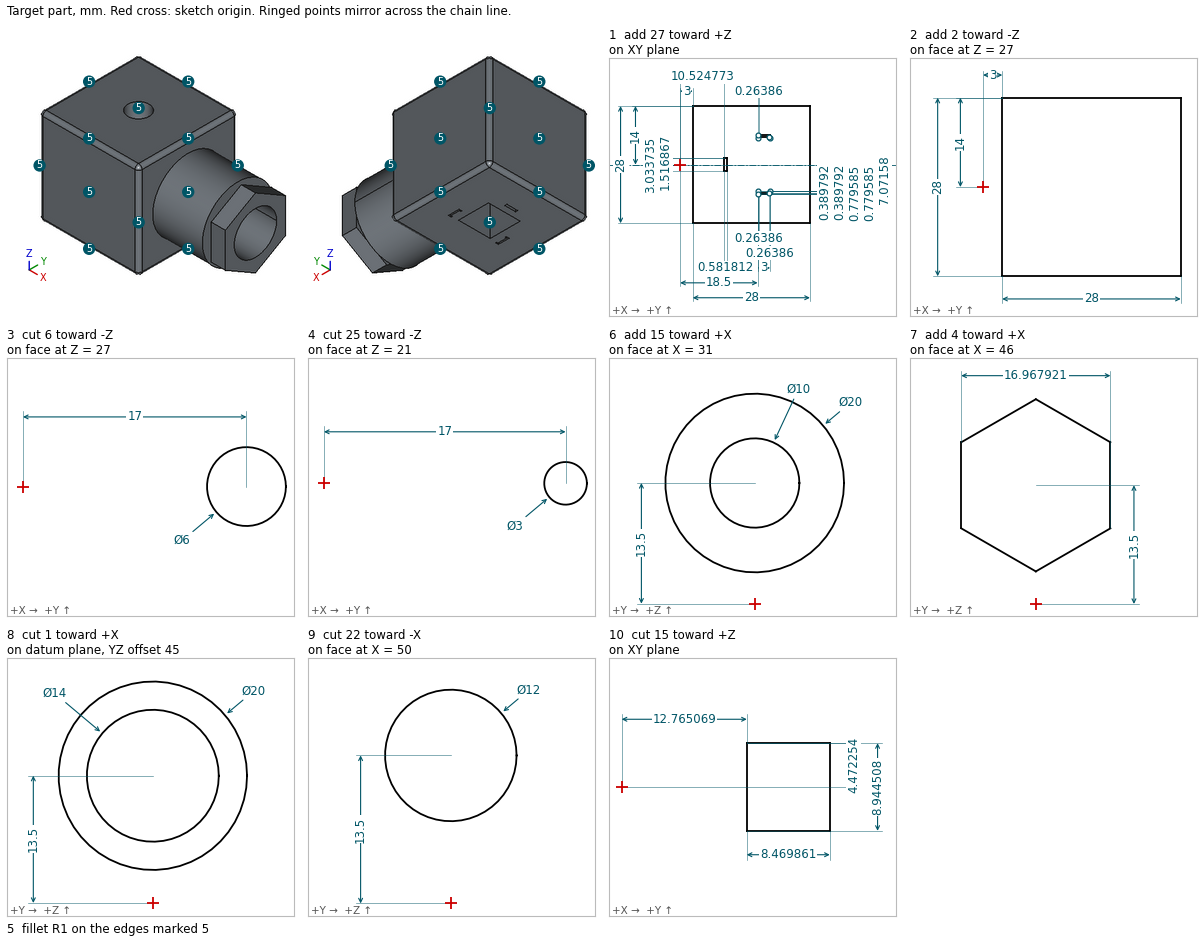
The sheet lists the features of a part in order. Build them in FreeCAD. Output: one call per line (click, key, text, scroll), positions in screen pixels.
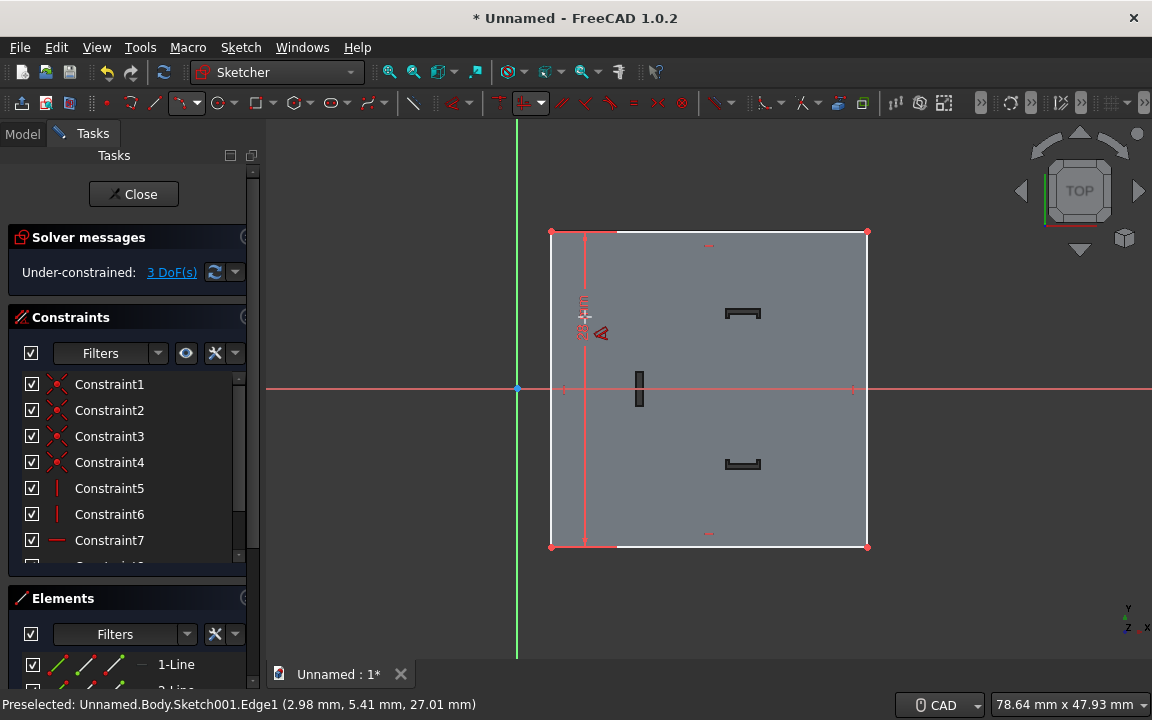
click(646, 547)
click(709, 581)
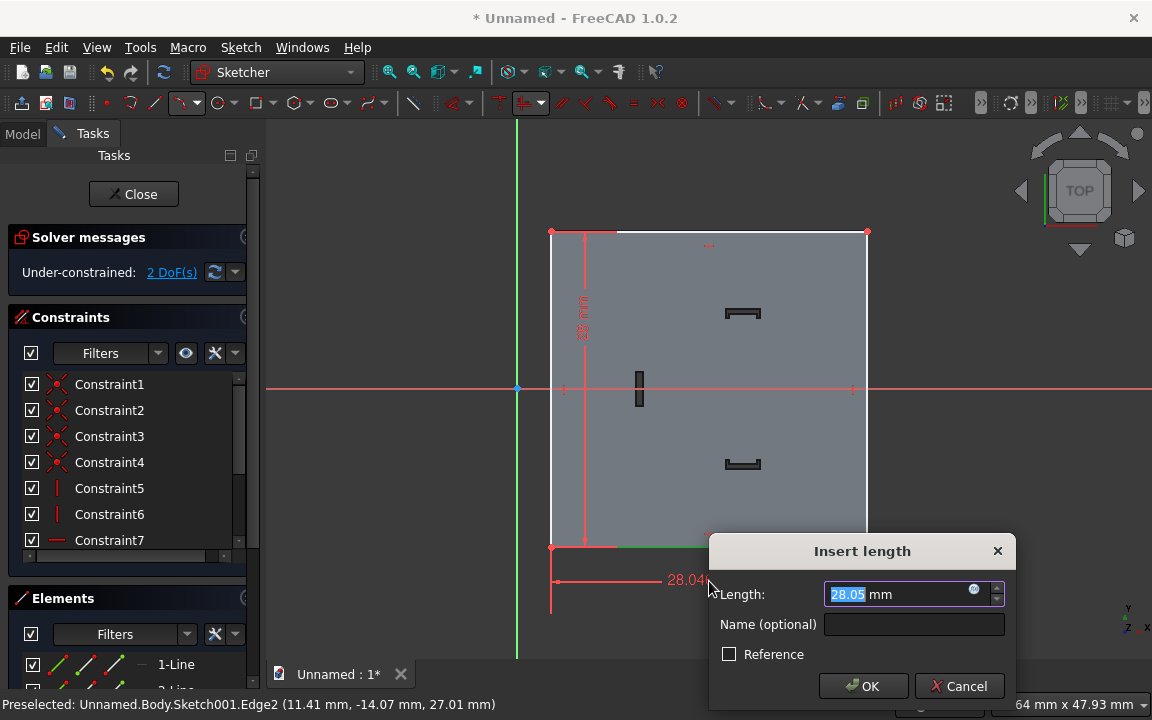
text(28)
key(Return)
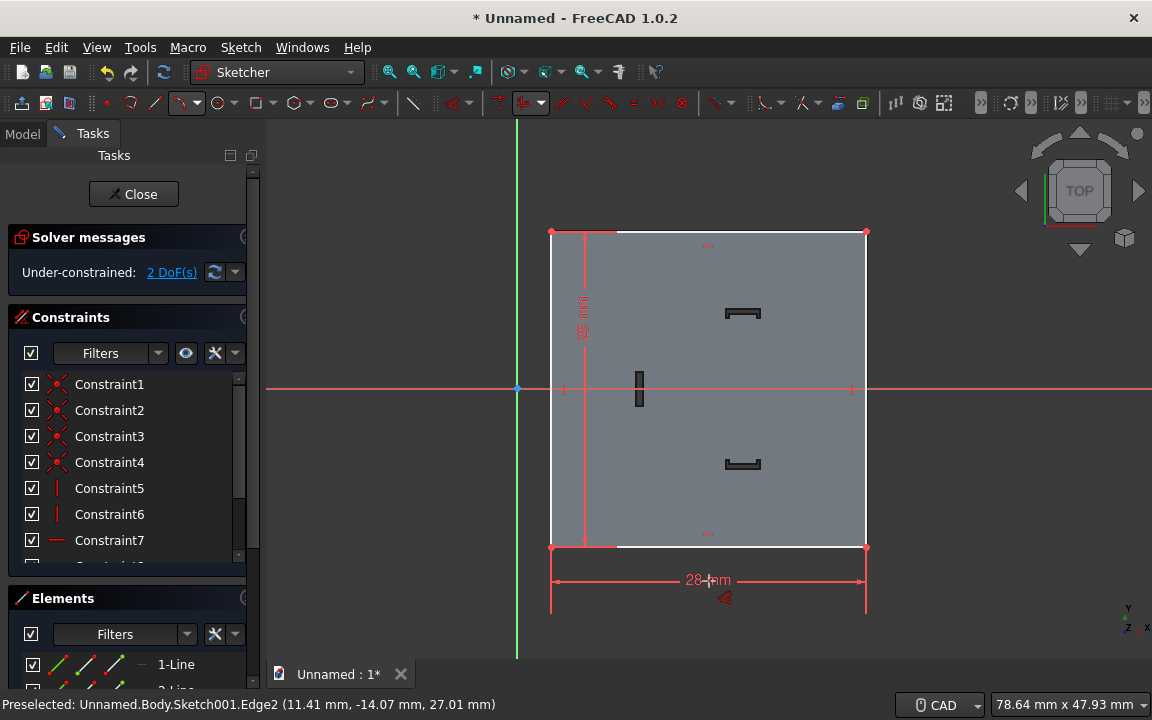
click(551, 232)
click(534, 198)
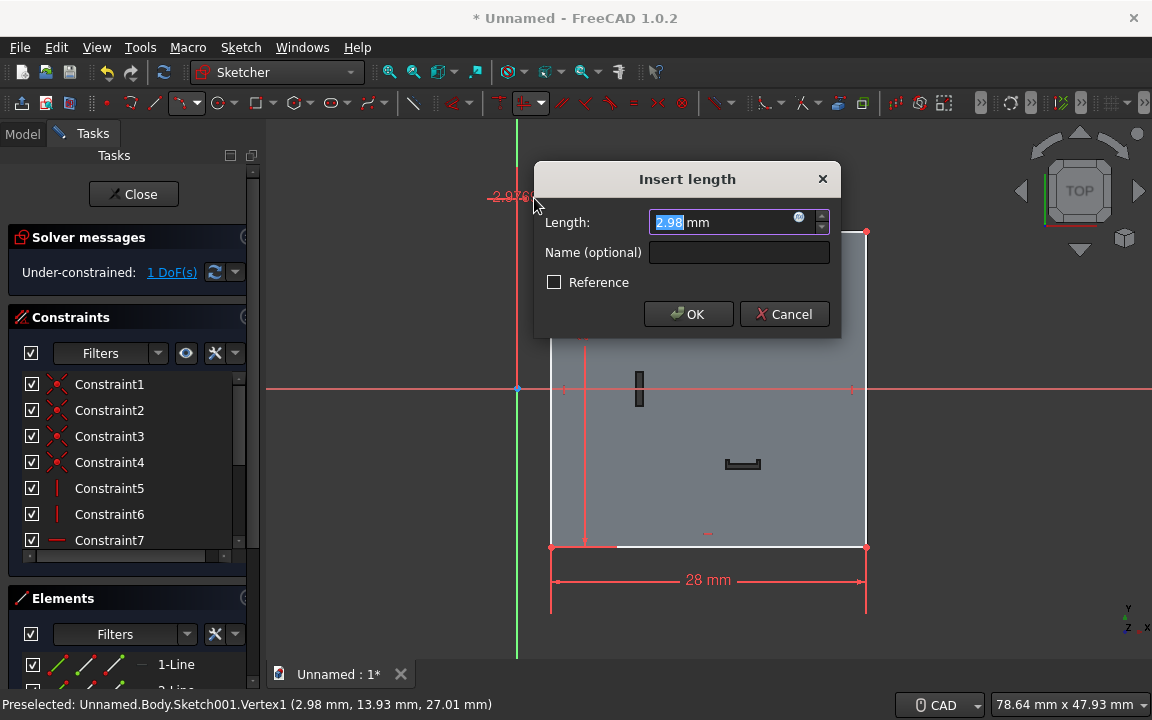
text(3)
key(Return)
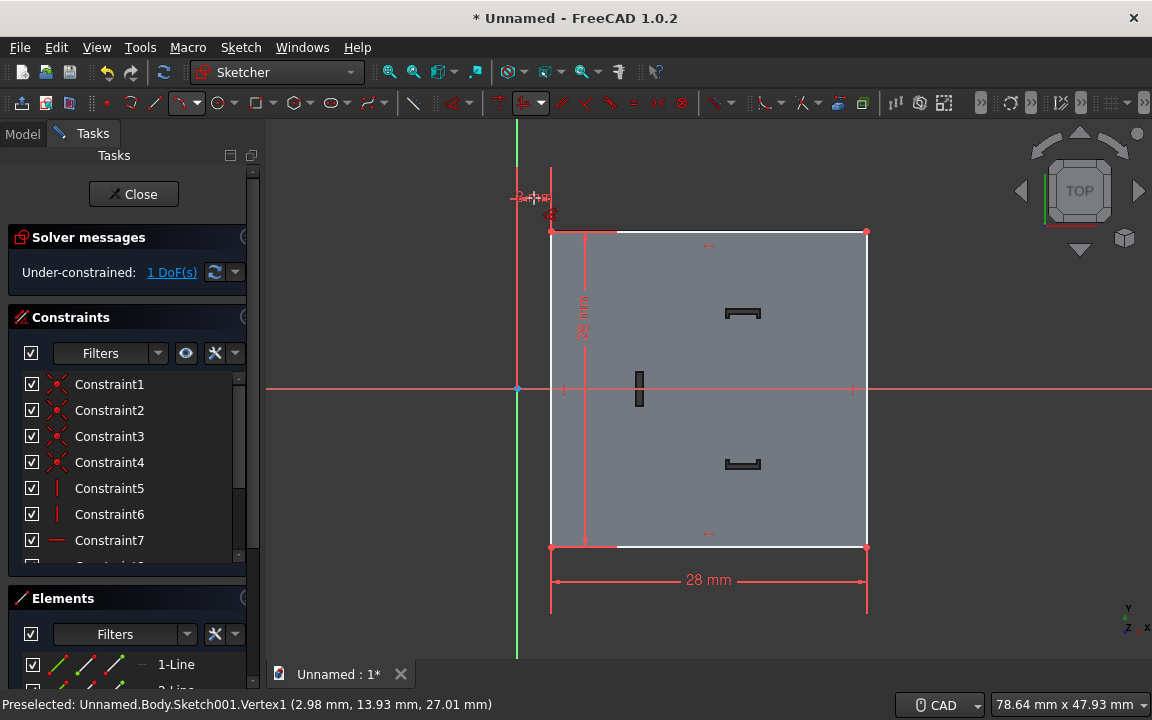
click(551, 232)
click(483, 310)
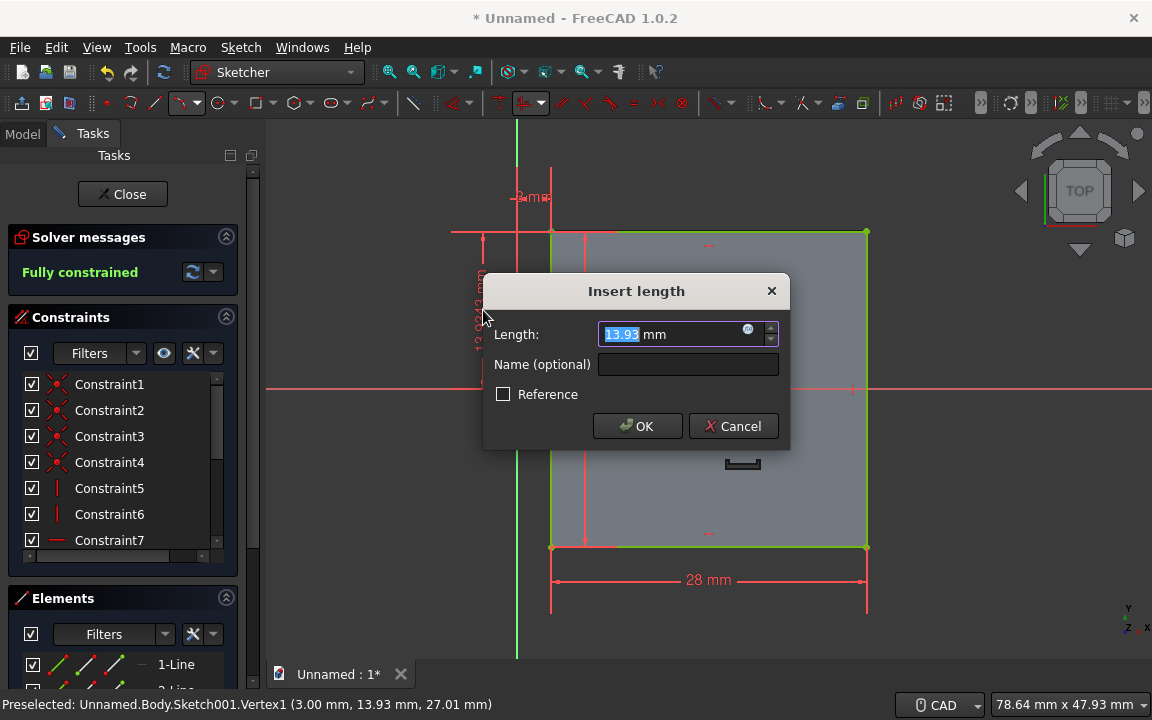
text(14)
key(Return)
key(Escape)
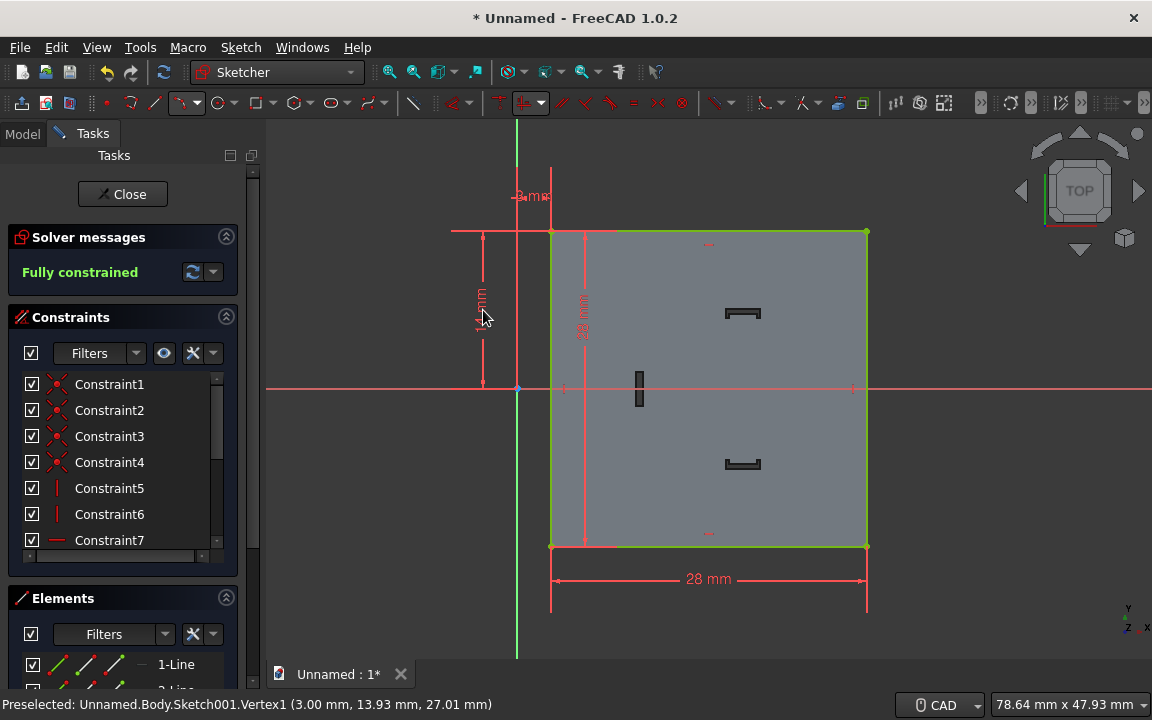
click(123, 194)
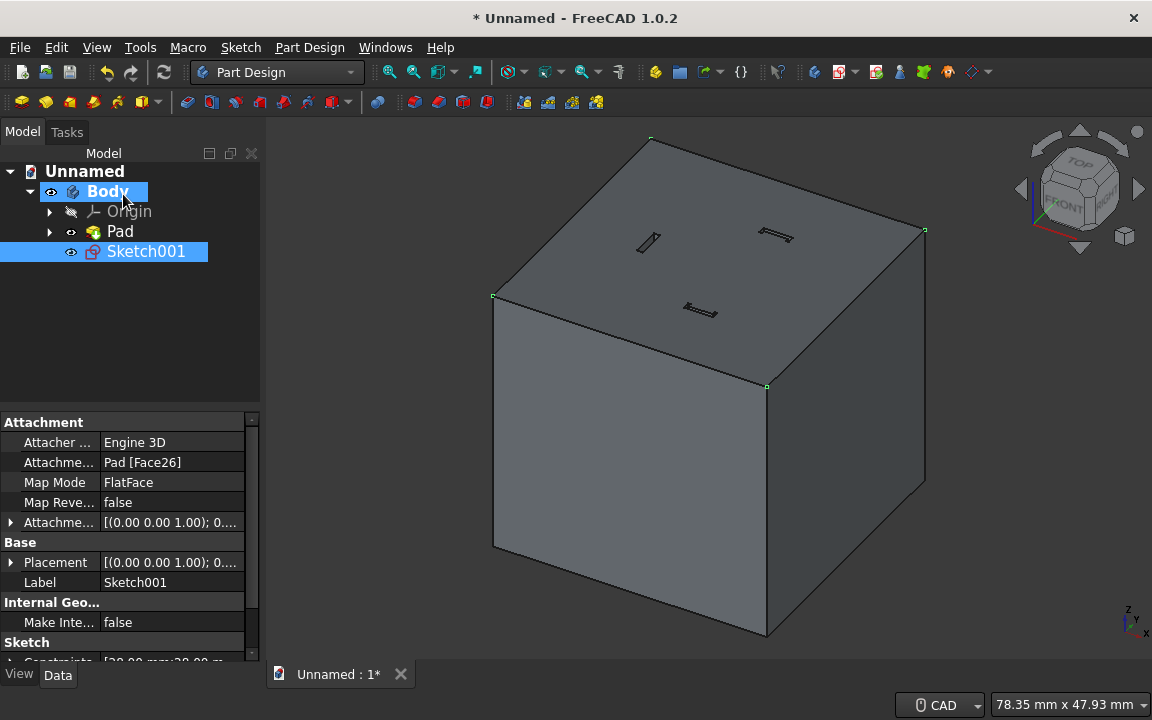
click(22, 102)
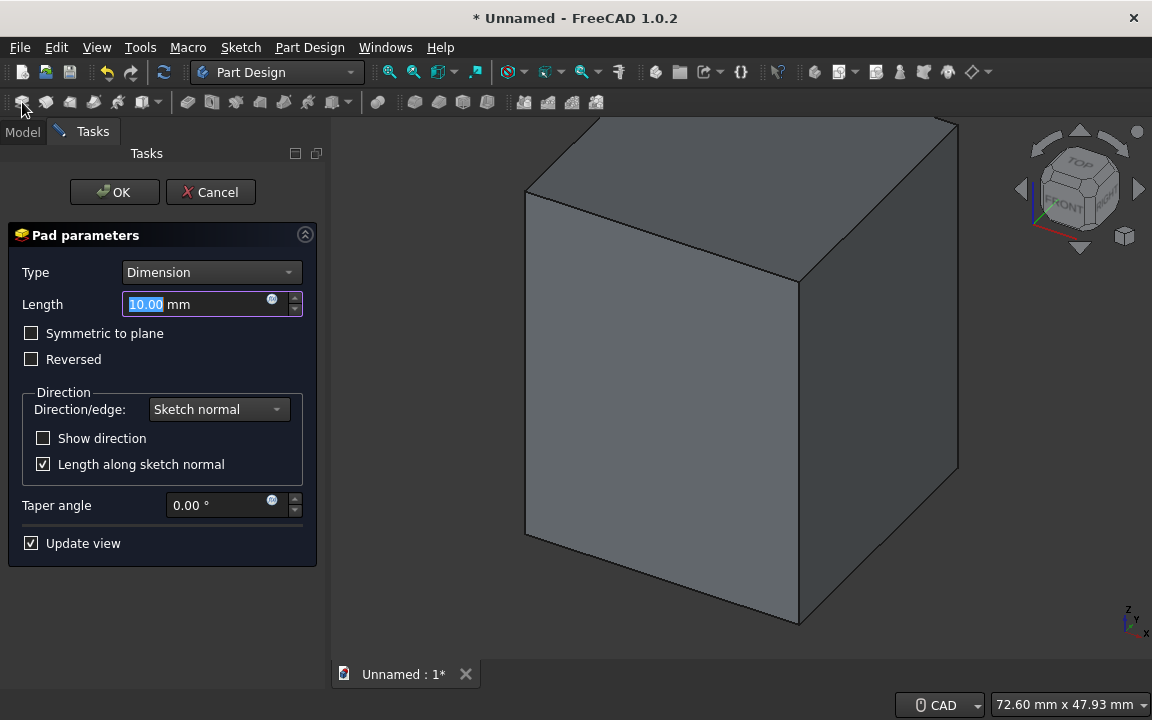
text(2)
key(Tab)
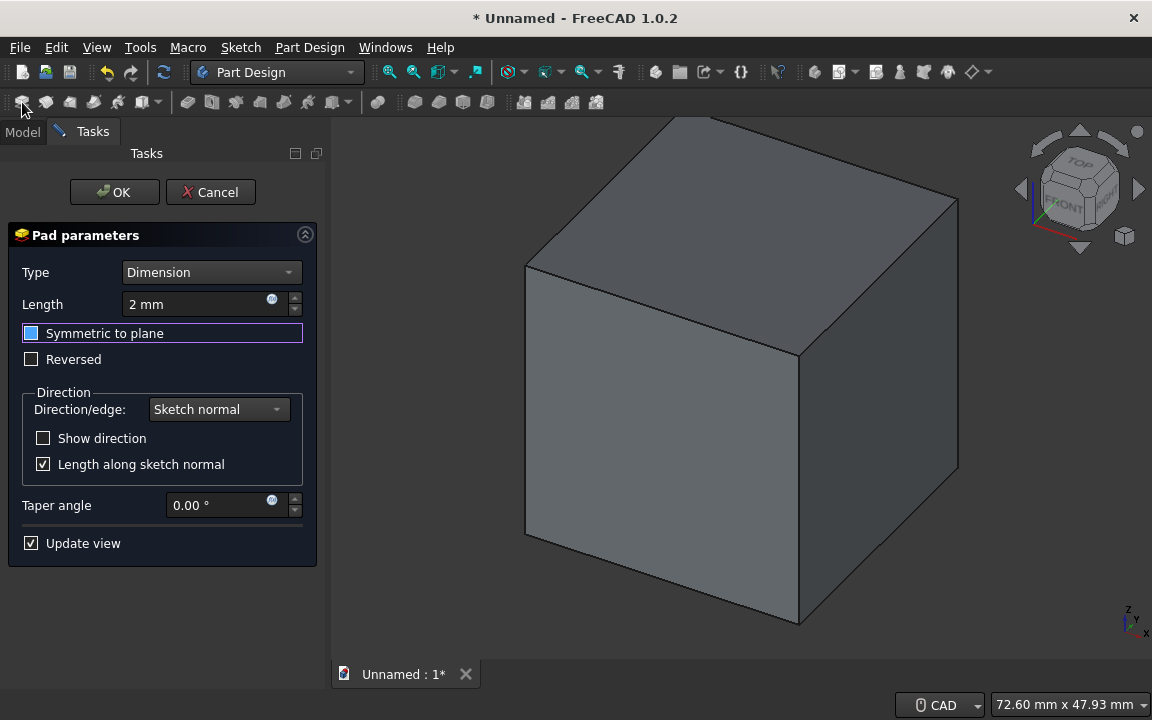
click(30, 359)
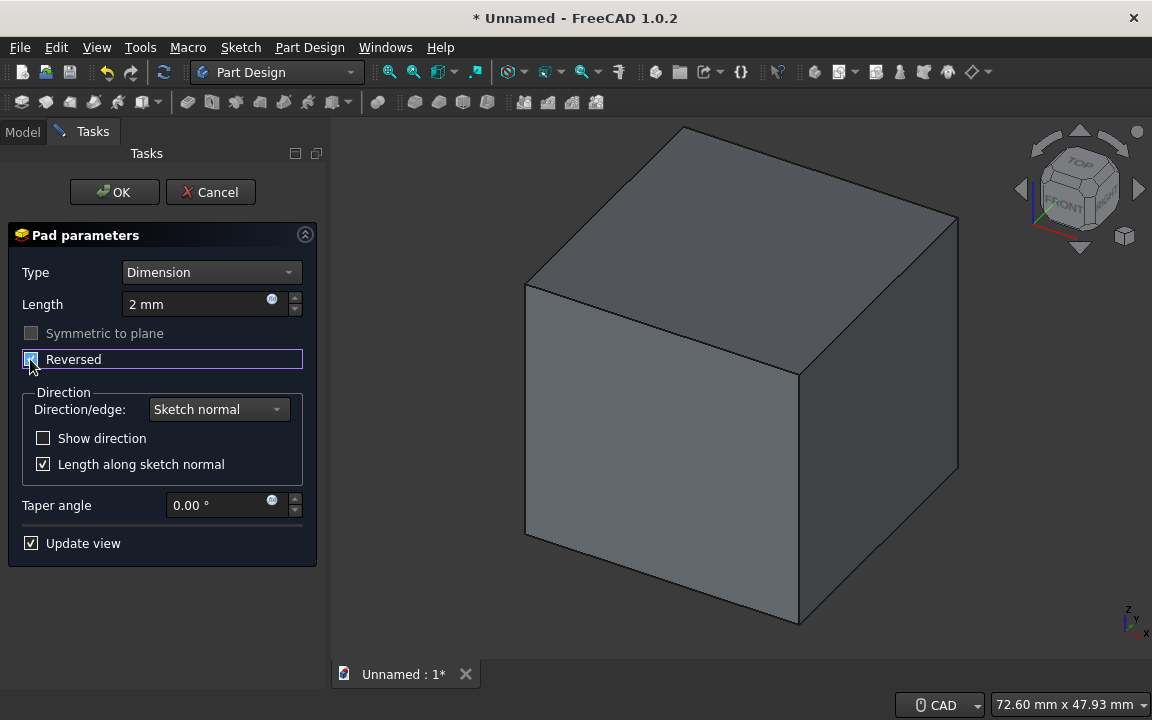
click(115, 192)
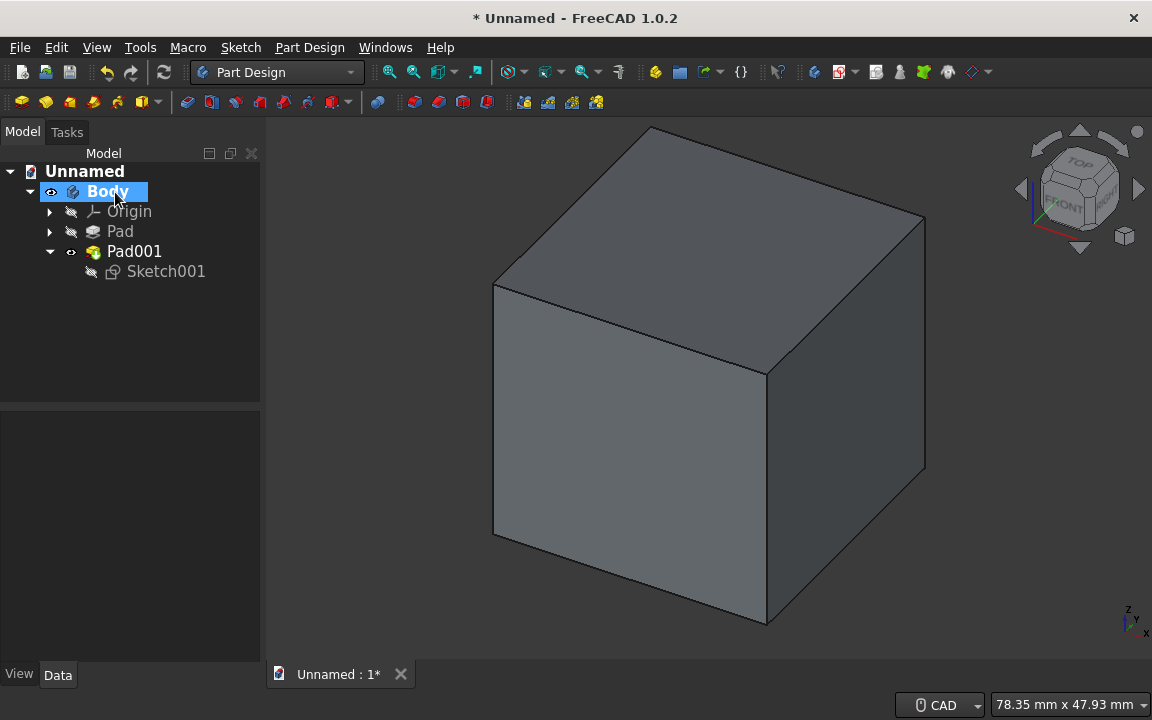
click(709, 250)